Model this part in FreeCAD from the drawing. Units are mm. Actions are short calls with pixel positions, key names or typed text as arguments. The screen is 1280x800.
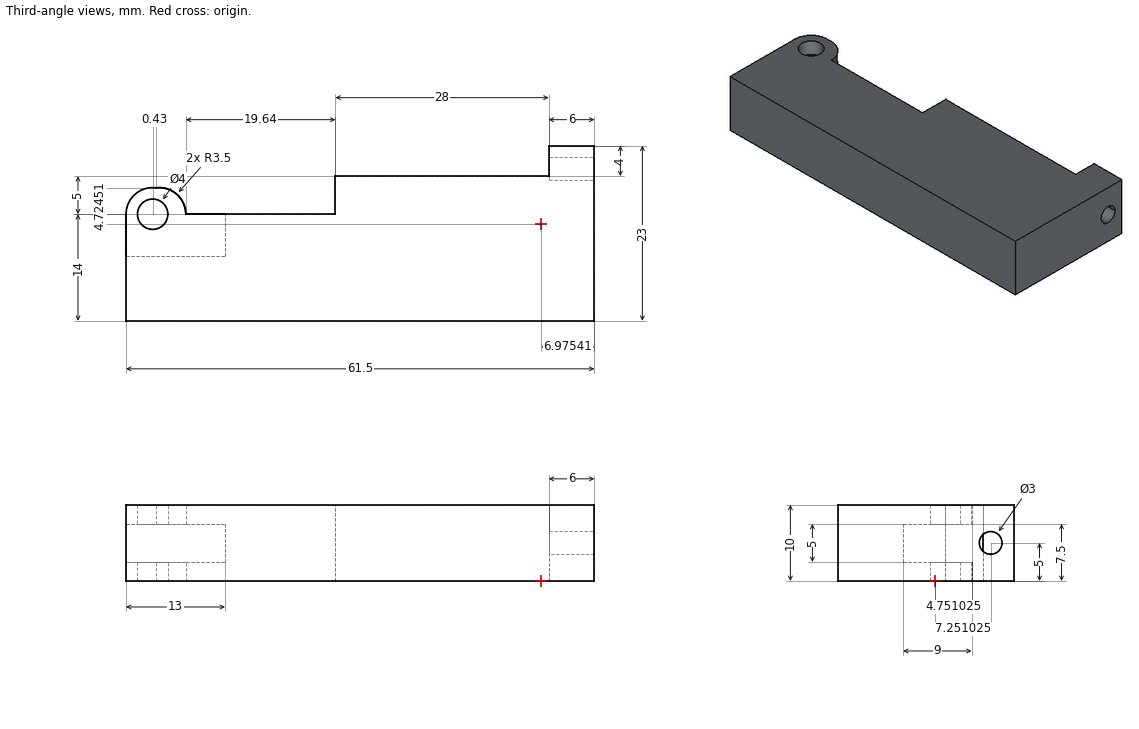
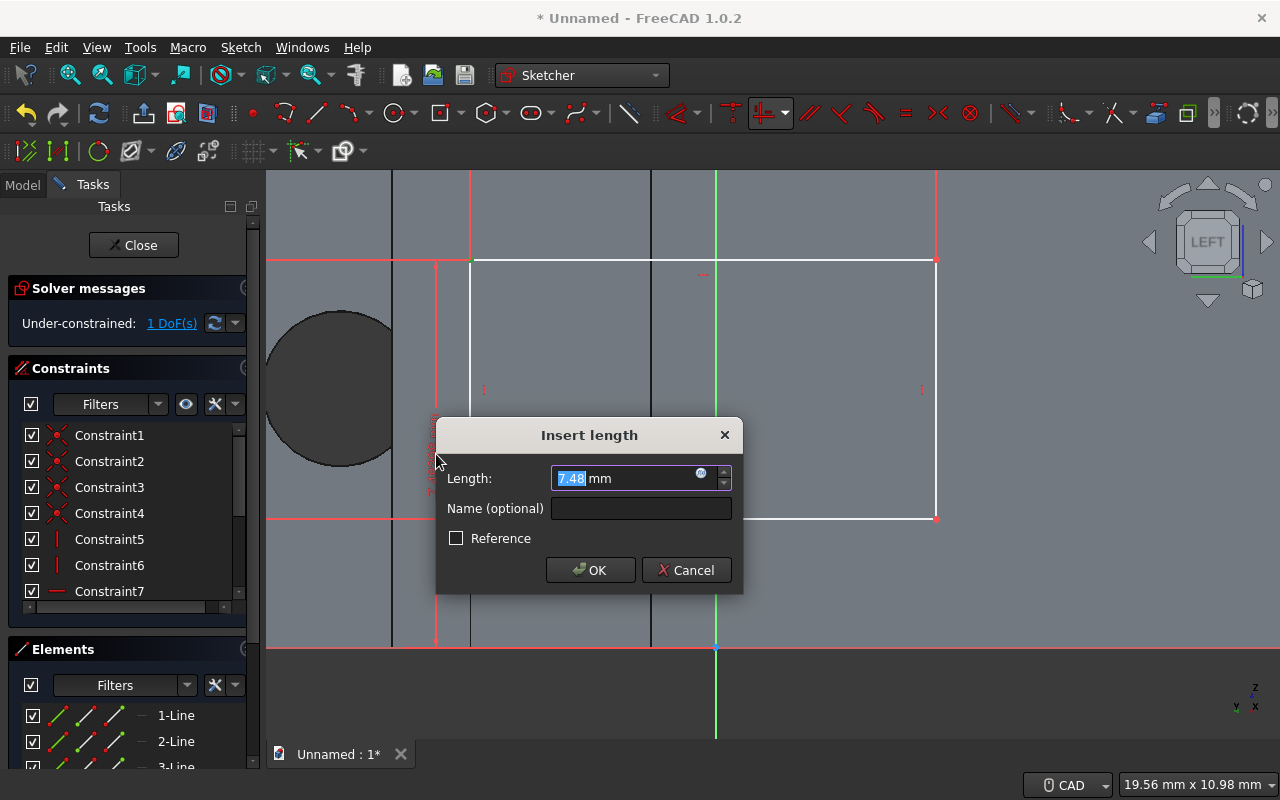
text(7.5)
key(Return)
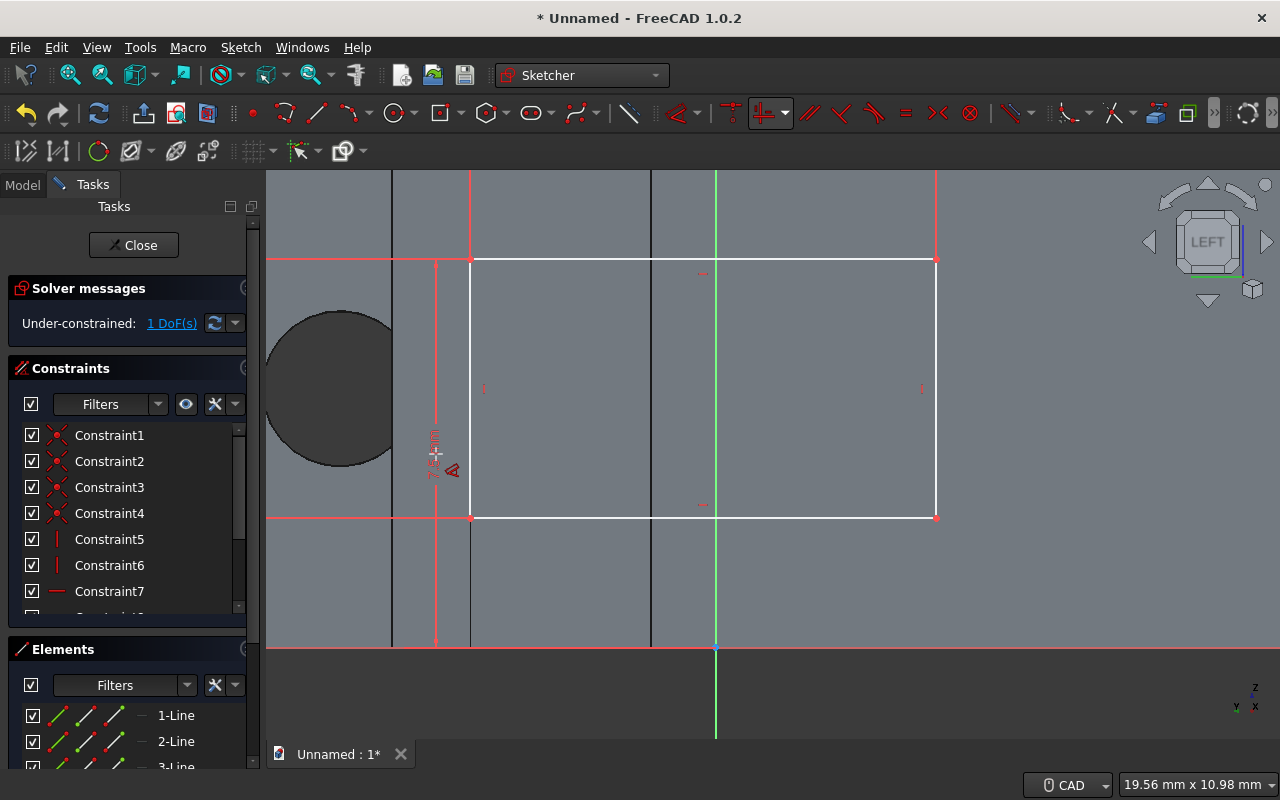
click(470, 259)
click(593, 682)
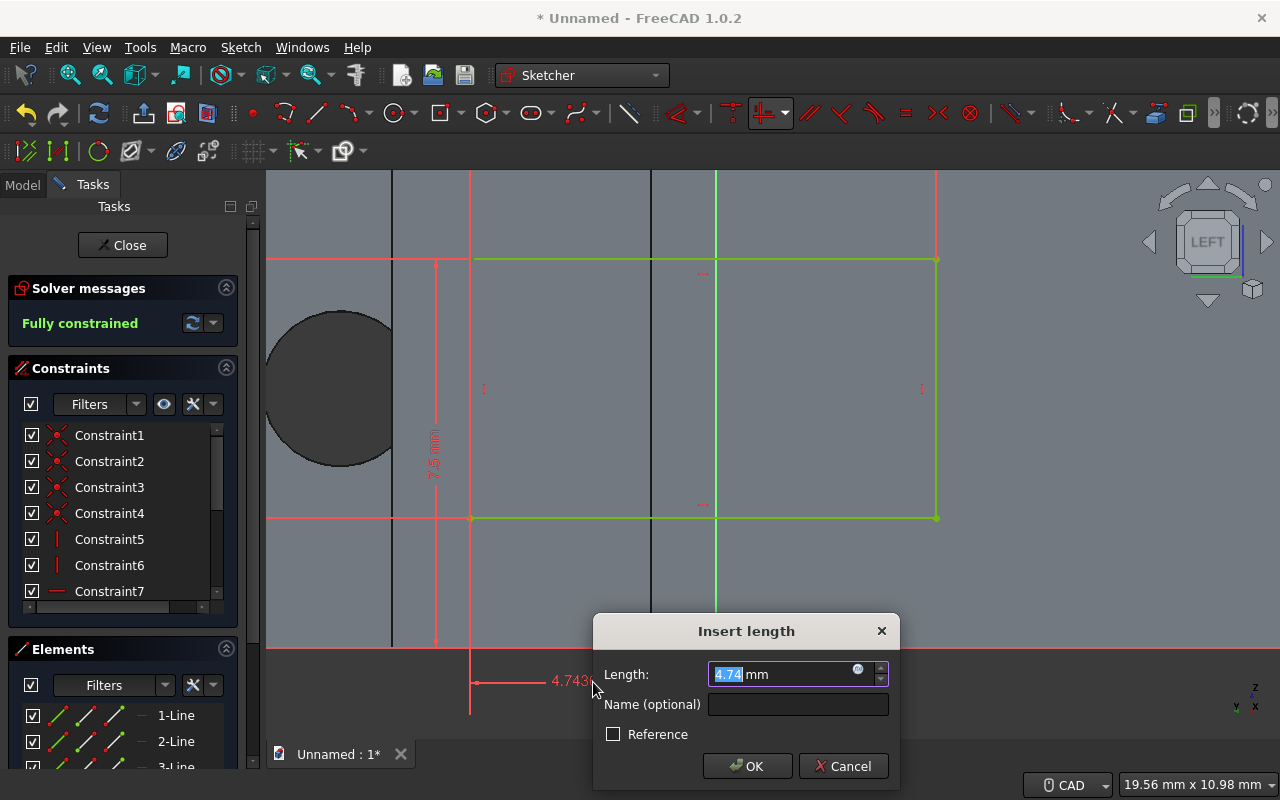
text(4.751025)
key(Return)
key(Escape)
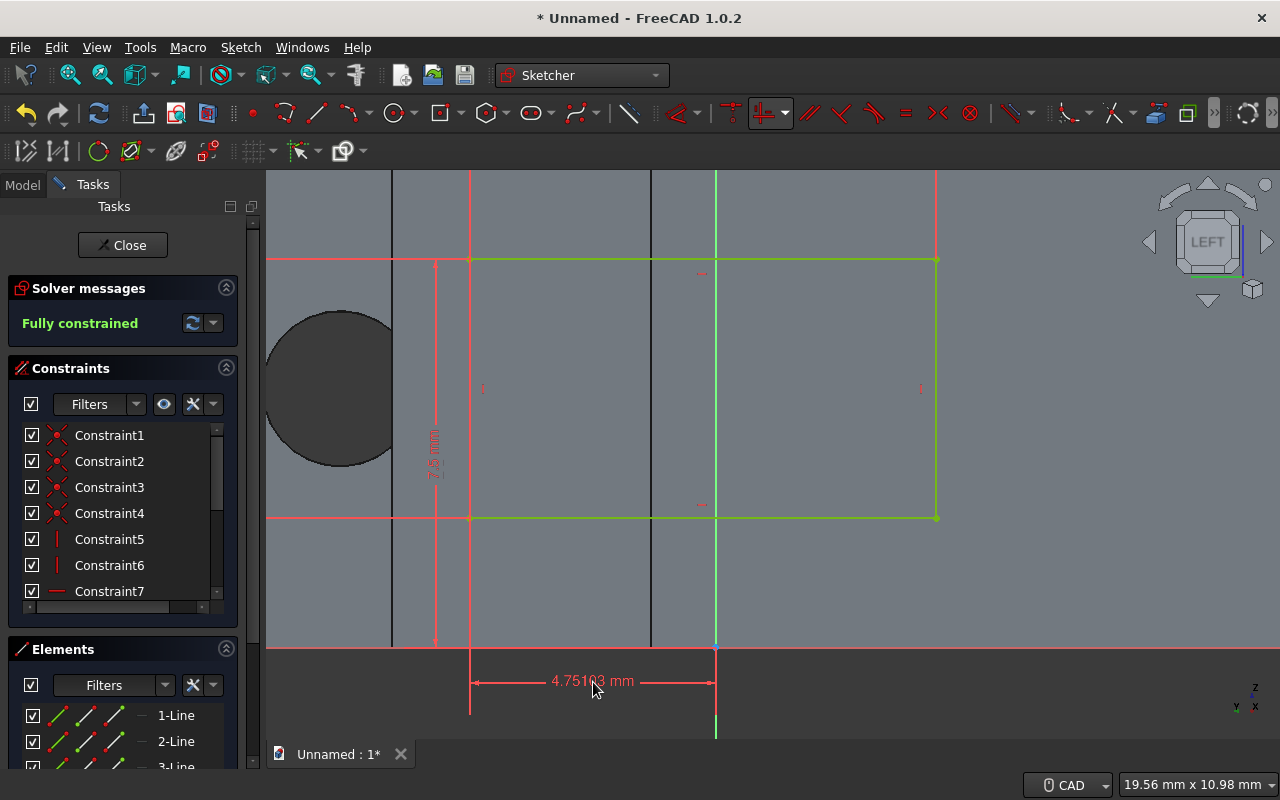
click(123, 245)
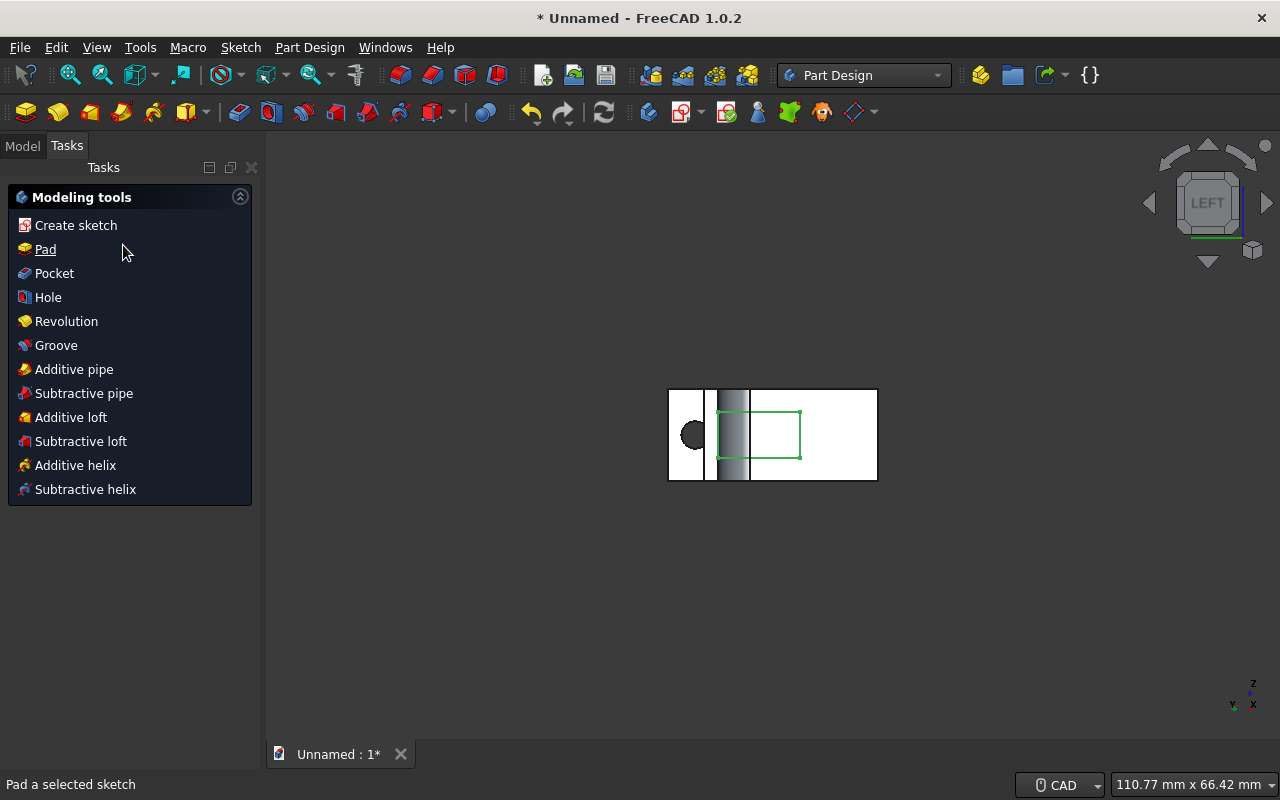
click(240, 112)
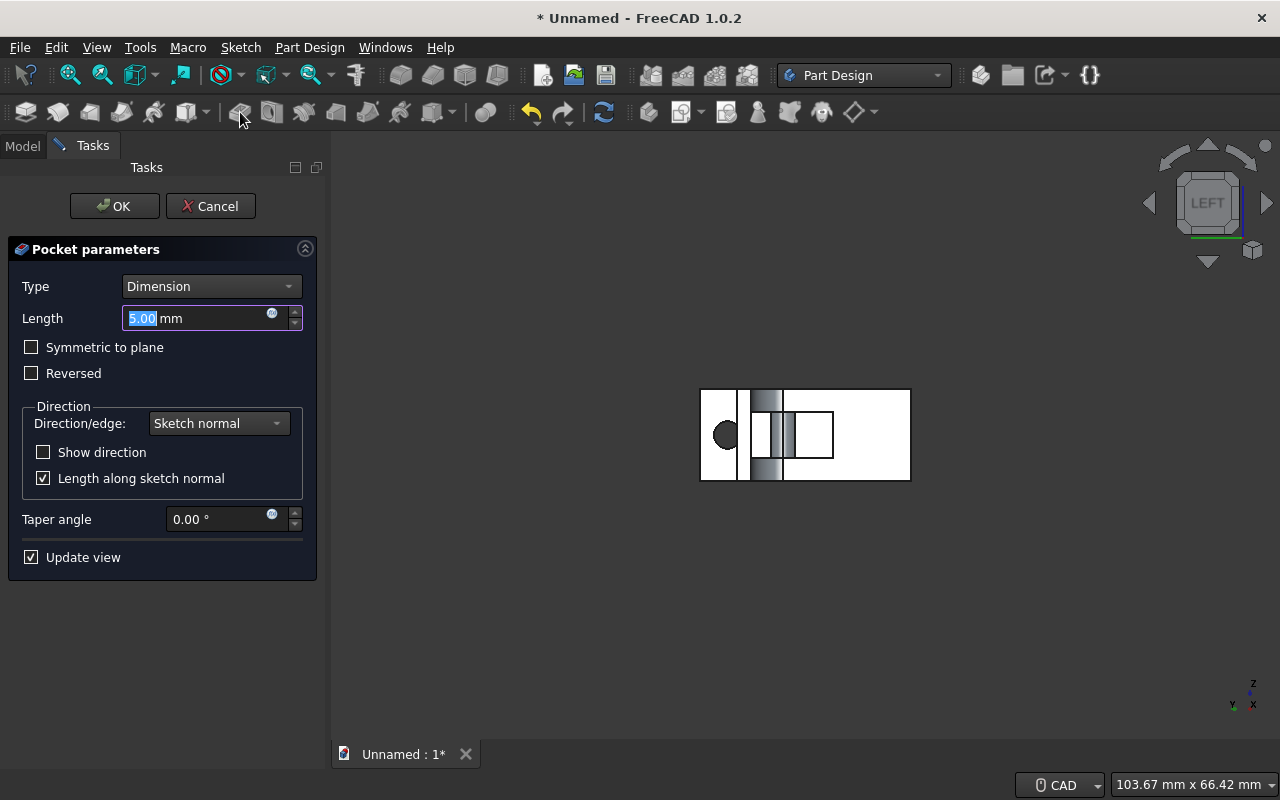
text(13)
key(Tab)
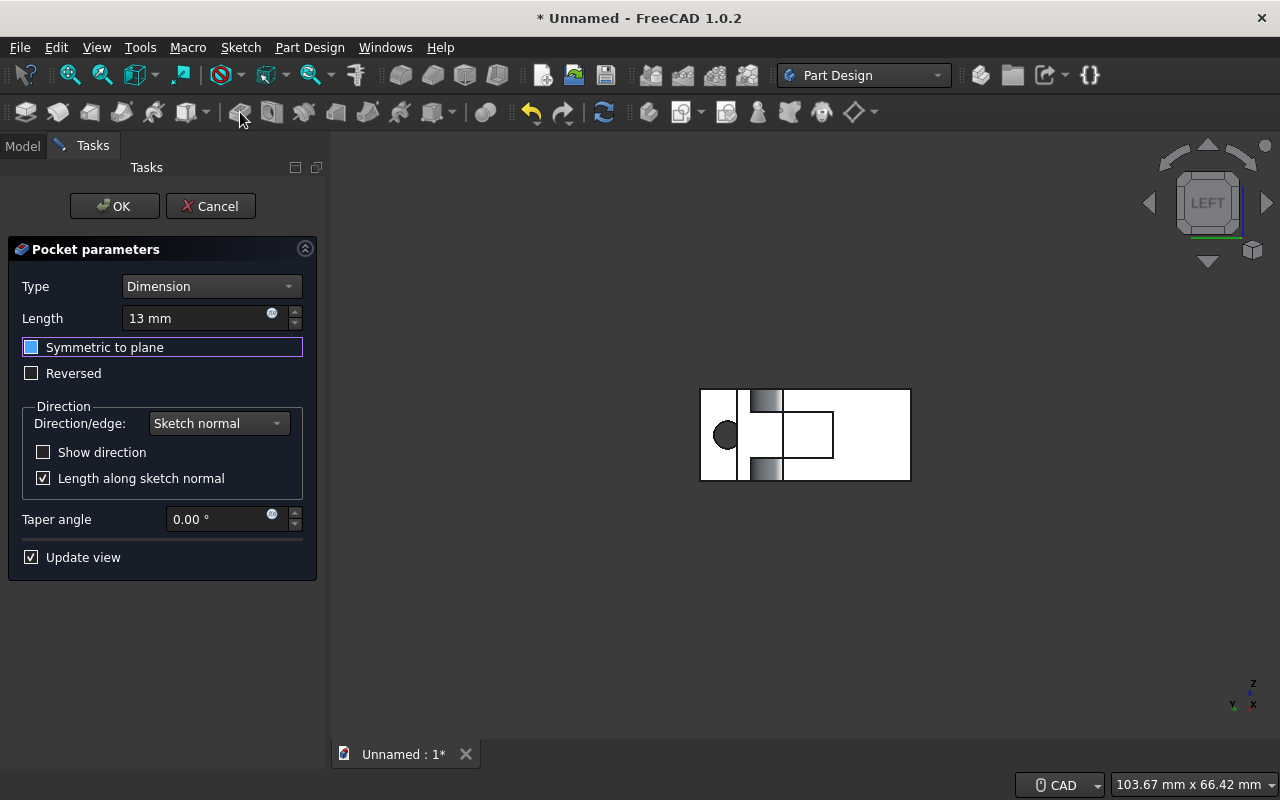
click(115, 206)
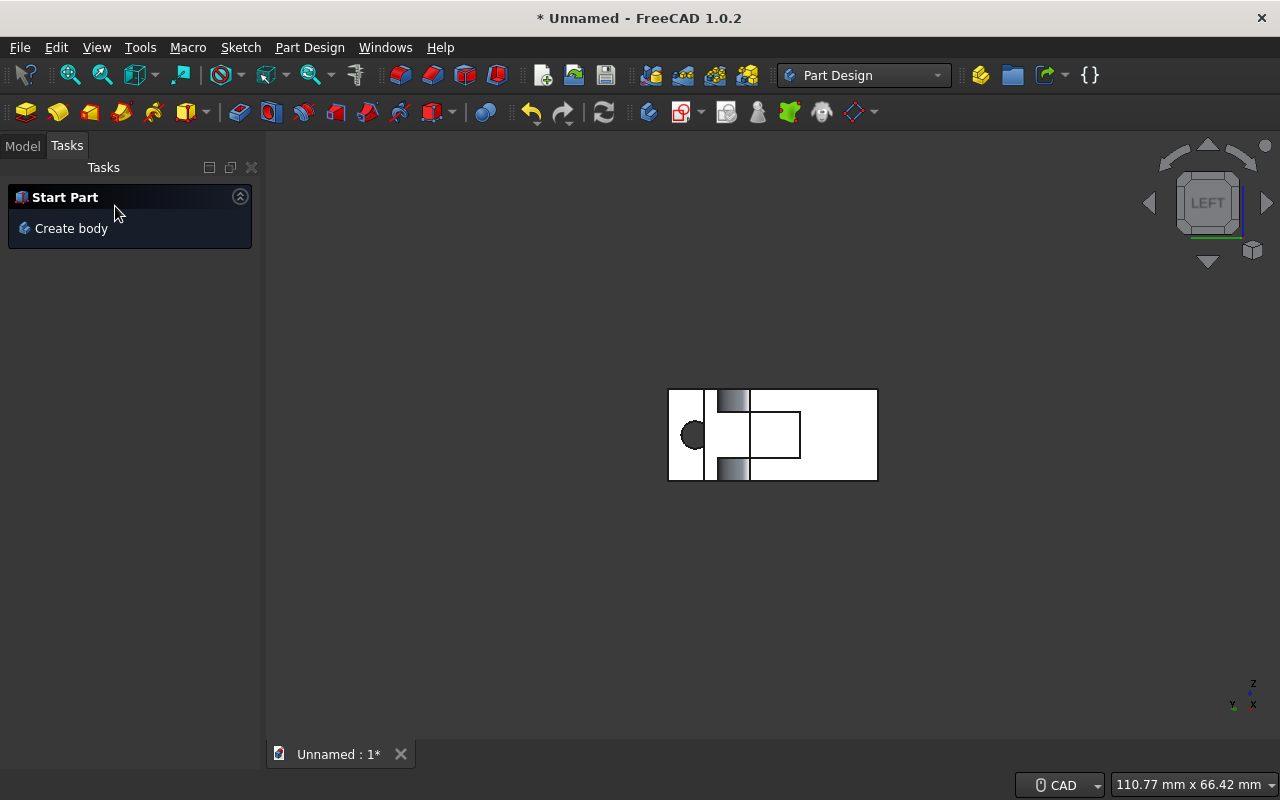
key(0)